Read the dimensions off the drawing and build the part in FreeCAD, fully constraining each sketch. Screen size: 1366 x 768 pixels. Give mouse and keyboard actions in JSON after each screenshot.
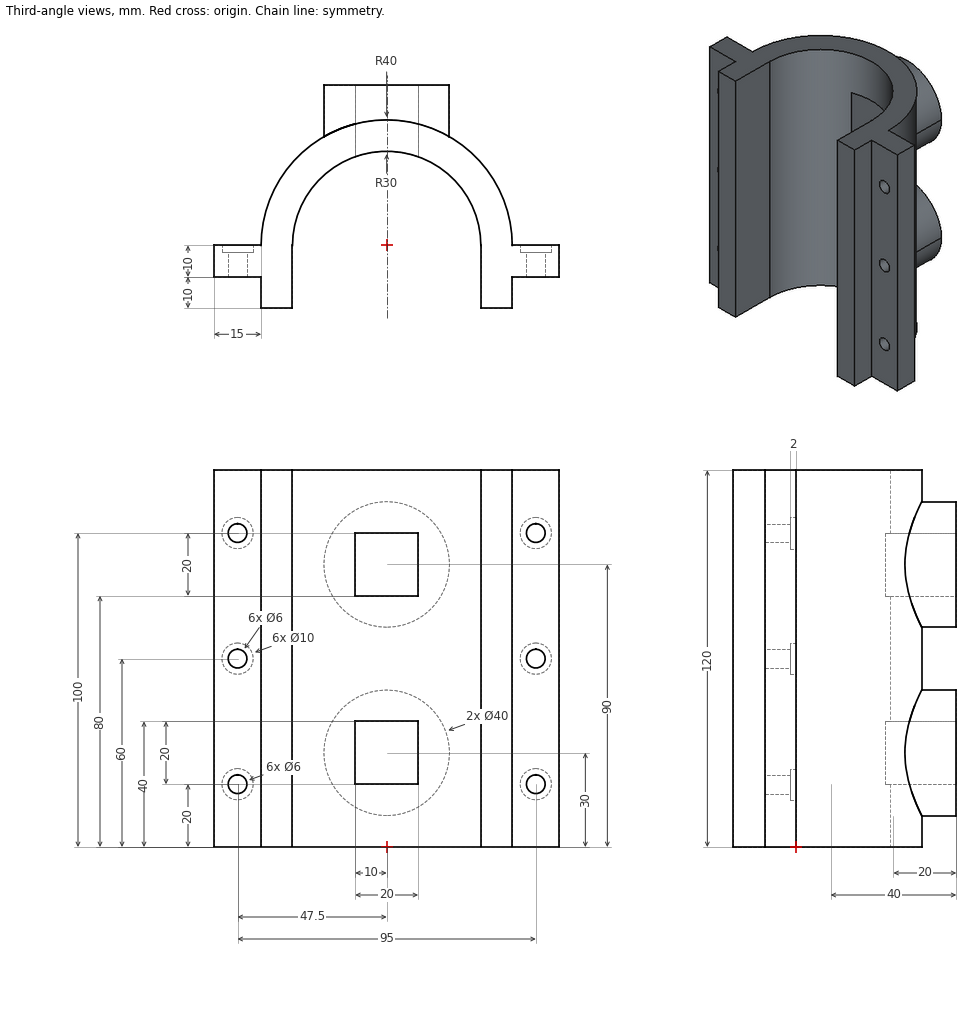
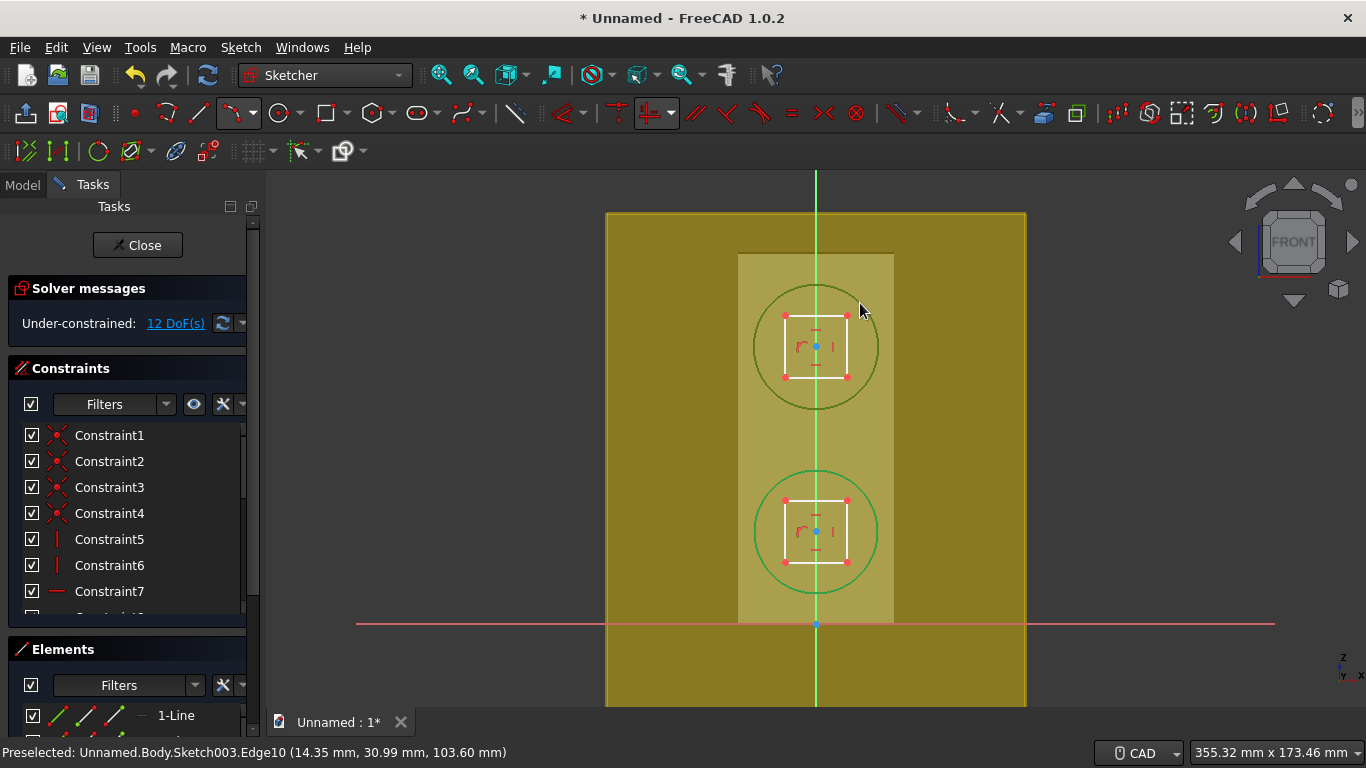
{"action": "left_click", "coordinate": [792, 114]}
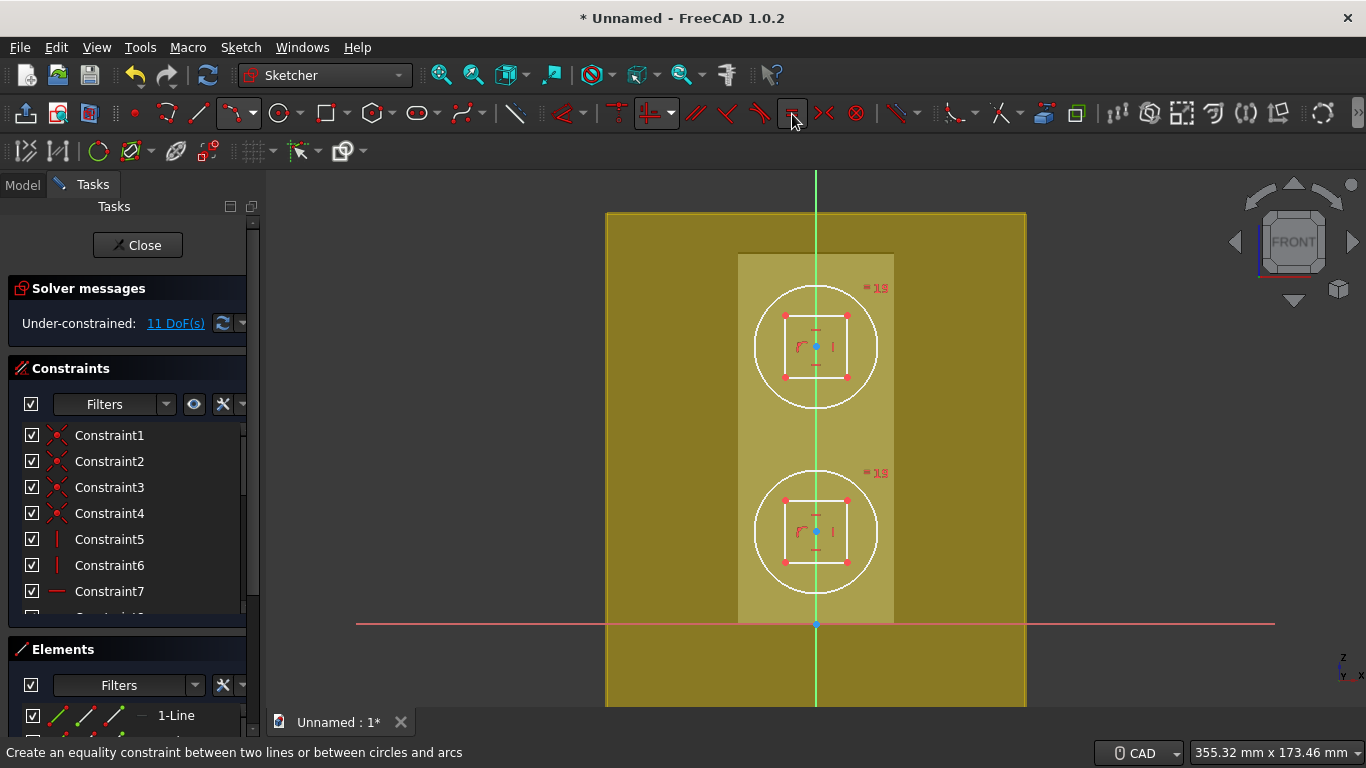
{"action": "left_click", "coordinate": [562, 114]}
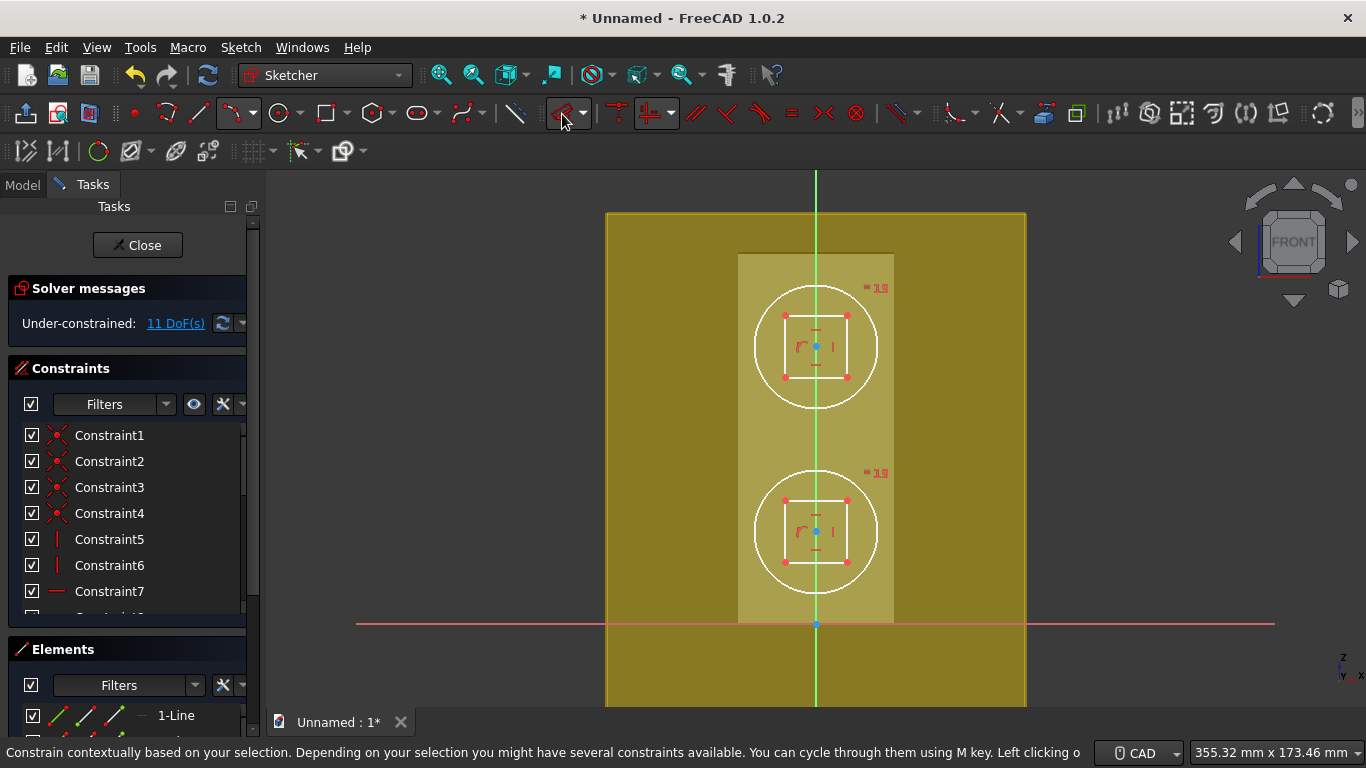
{"action": "left_click", "coordinate": [859, 488]}
{"action": "left_click", "coordinate": [881, 465]}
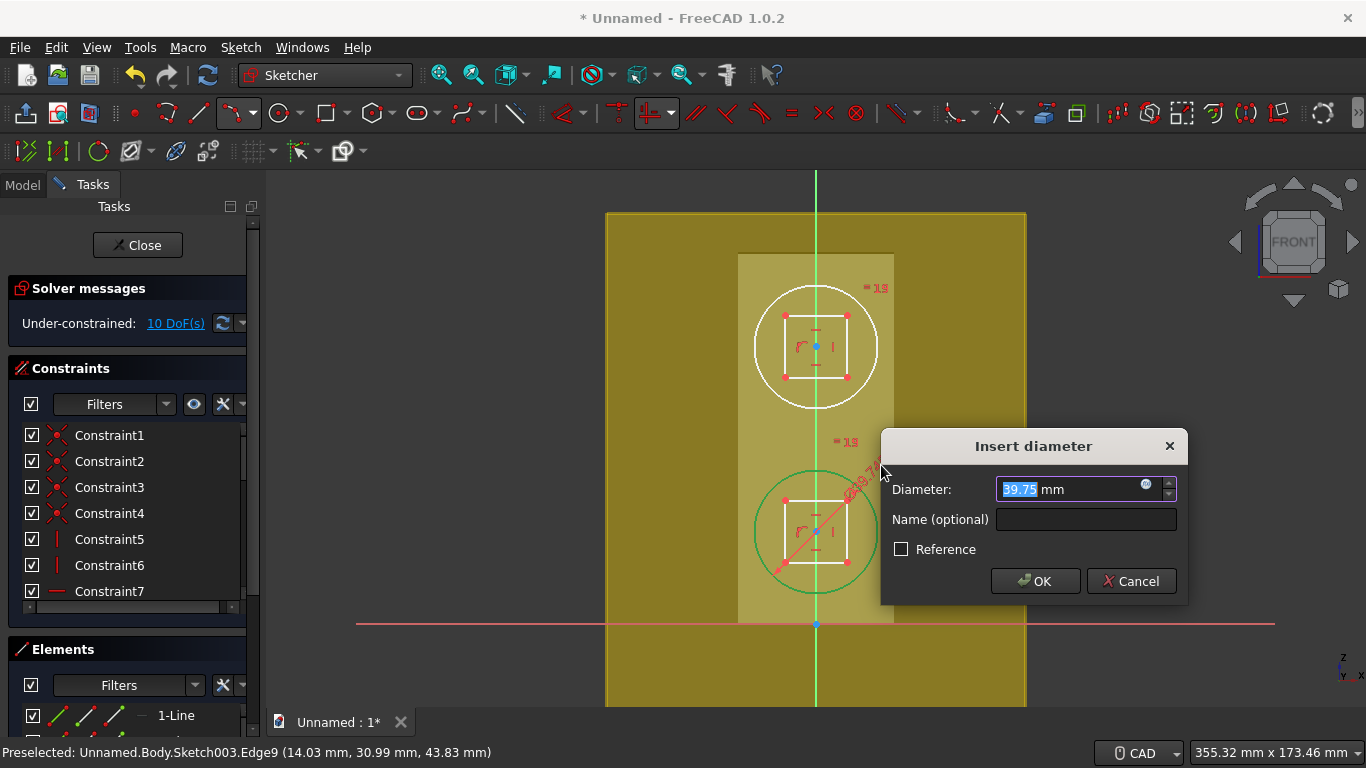
{"action": "type", "text": "40"}
{"action": "key", "text": "Return"}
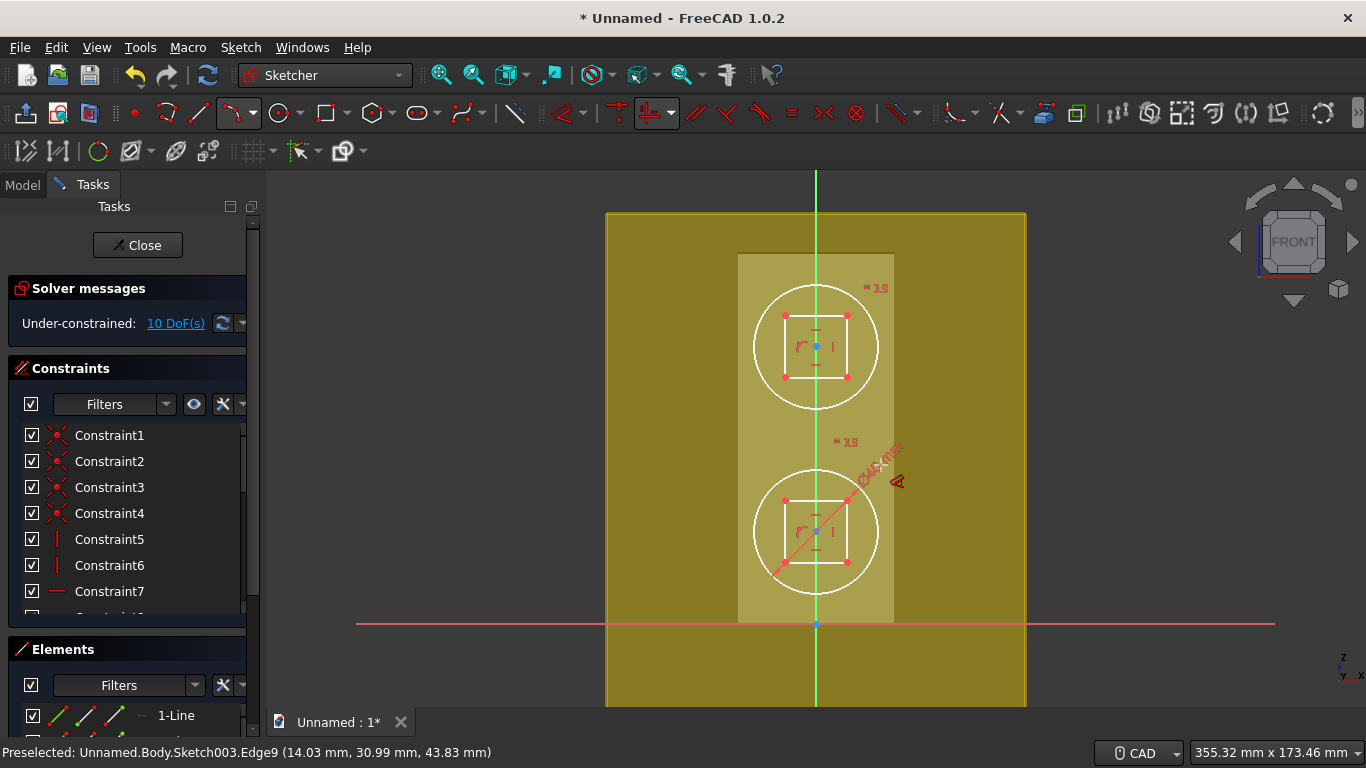
{"action": "left_click", "coordinate": [785, 520]}
{"action": "left_click", "coordinate": [727, 532]}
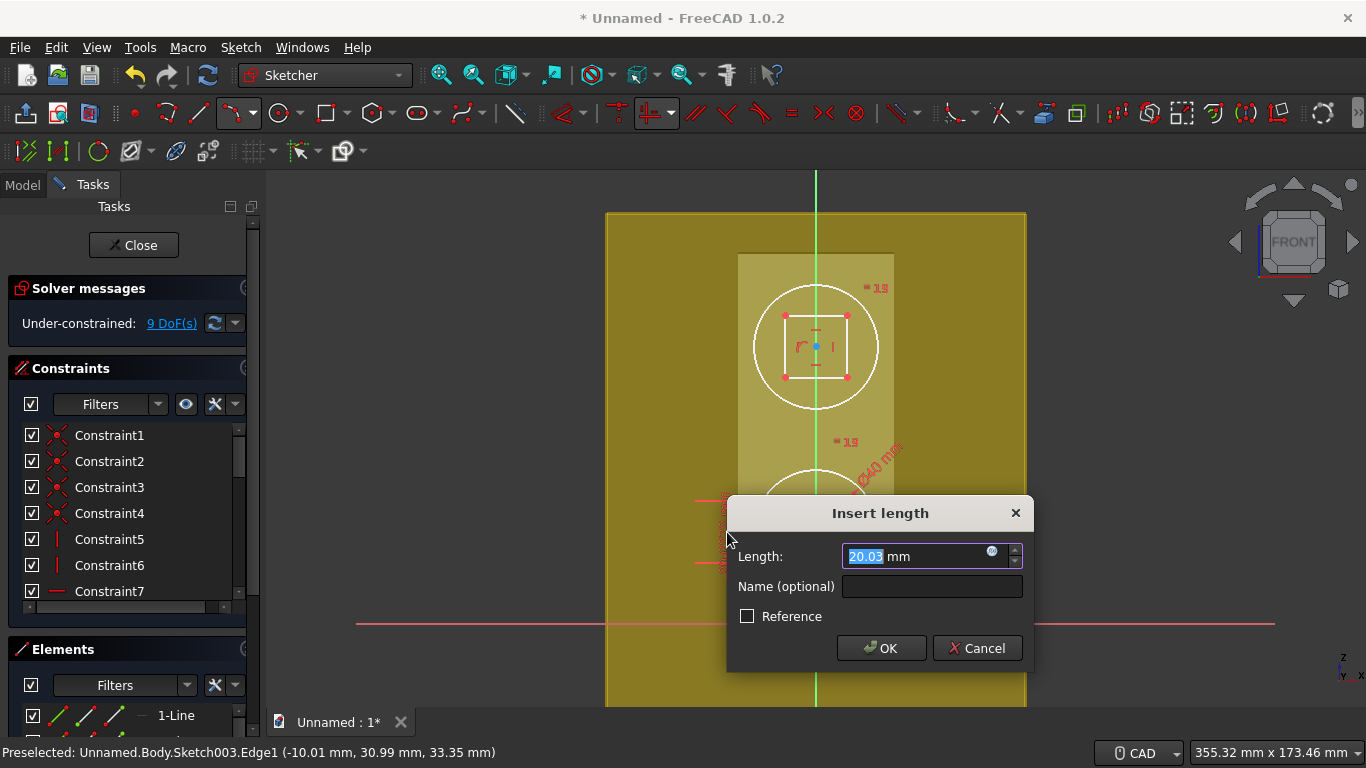
{"action": "type", "text": "20"}
{"action": "key", "text": "Return"}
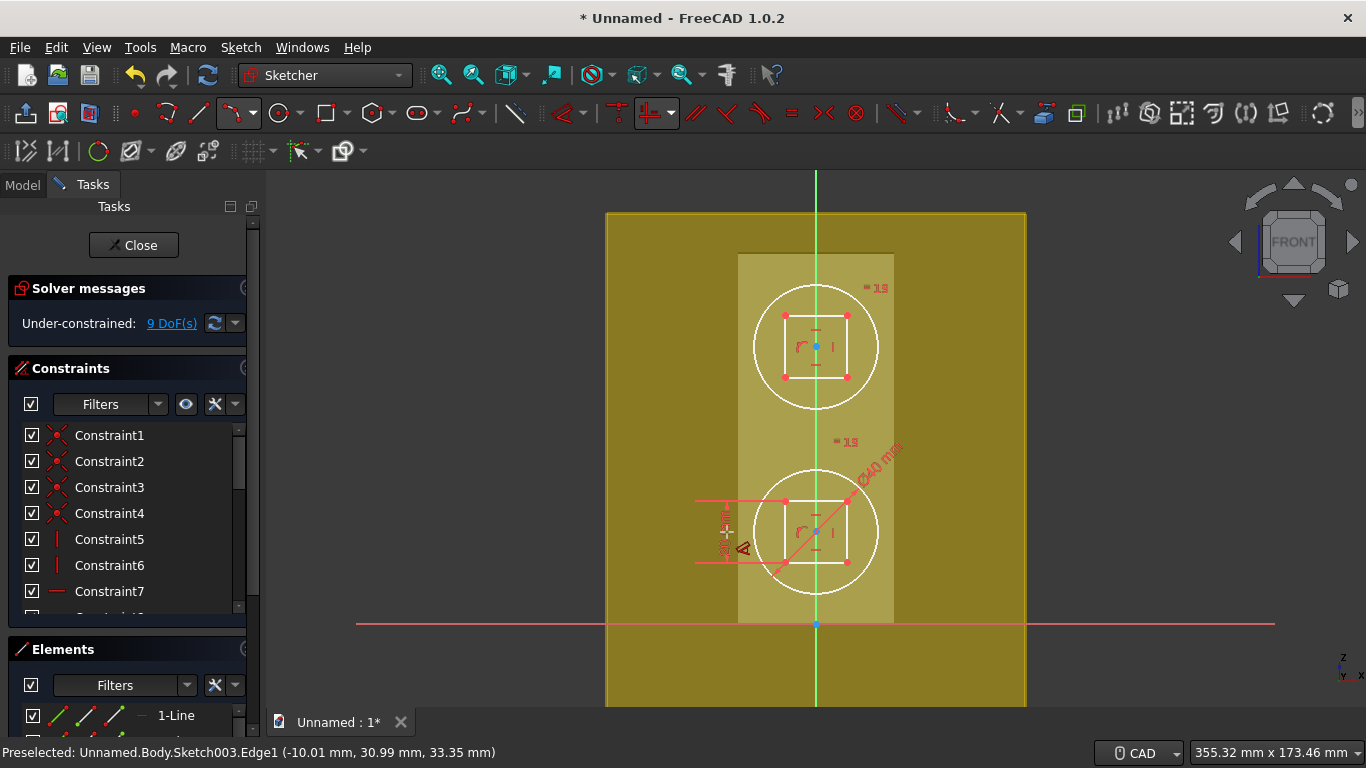
{"action": "left_click", "coordinate": [804, 563]}
{"action": "left_click", "coordinate": [802, 529]}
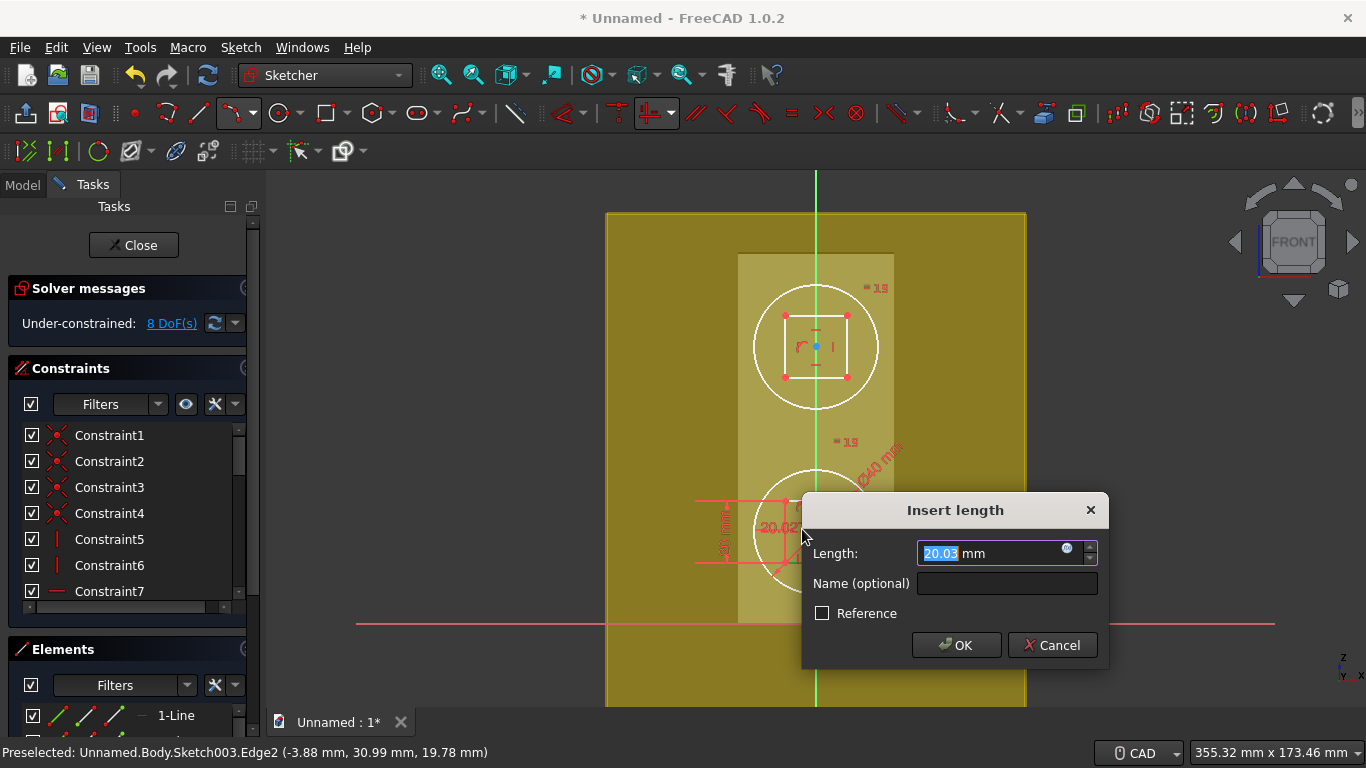
{"action": "type", "text": "20"}
{"action": "key", "text": "Return"}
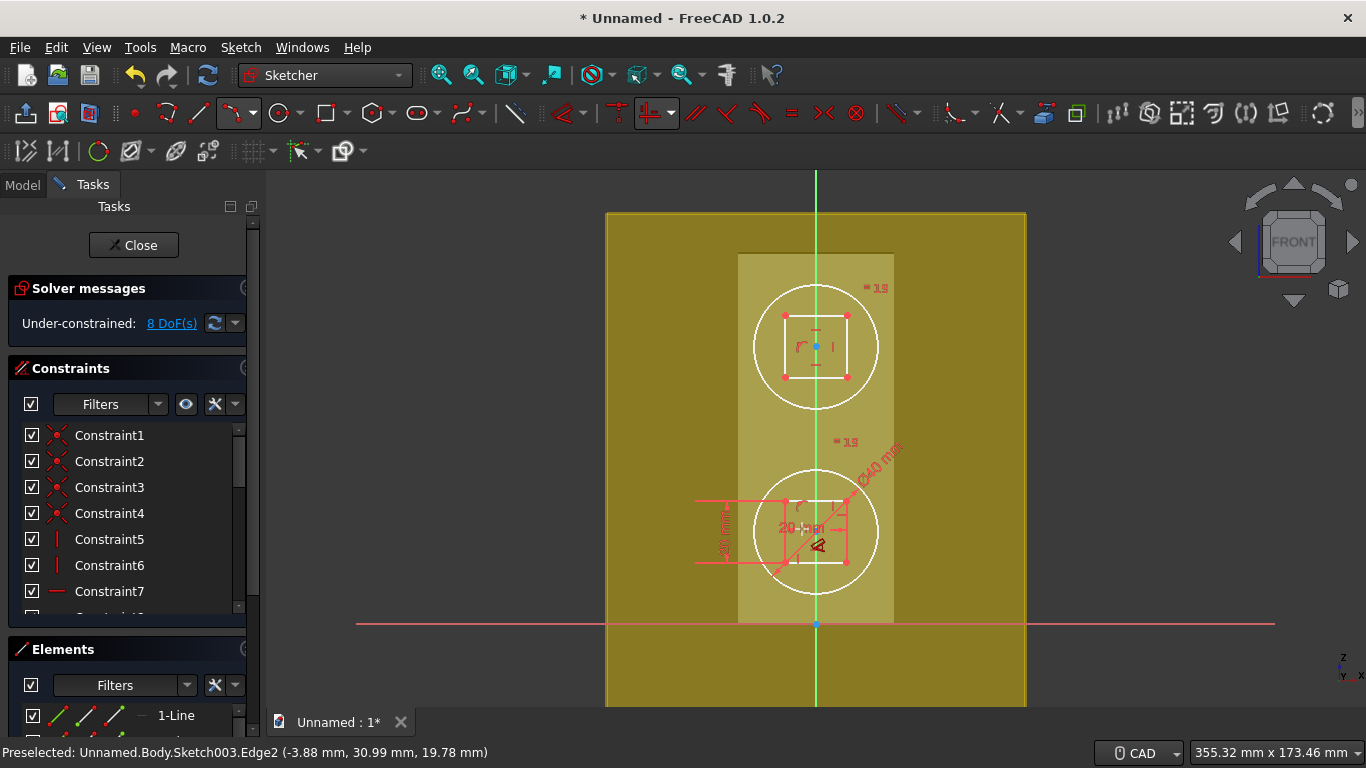
{"action": "left_click", "coordinate": [785, 335]}
{"action": "left_click", "coordinate": [727, 347]}